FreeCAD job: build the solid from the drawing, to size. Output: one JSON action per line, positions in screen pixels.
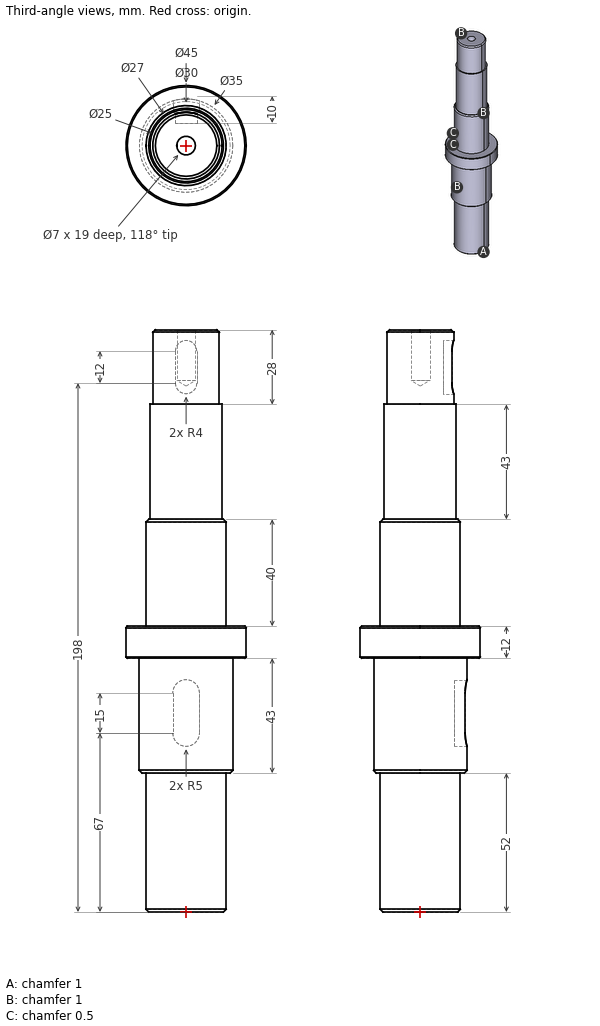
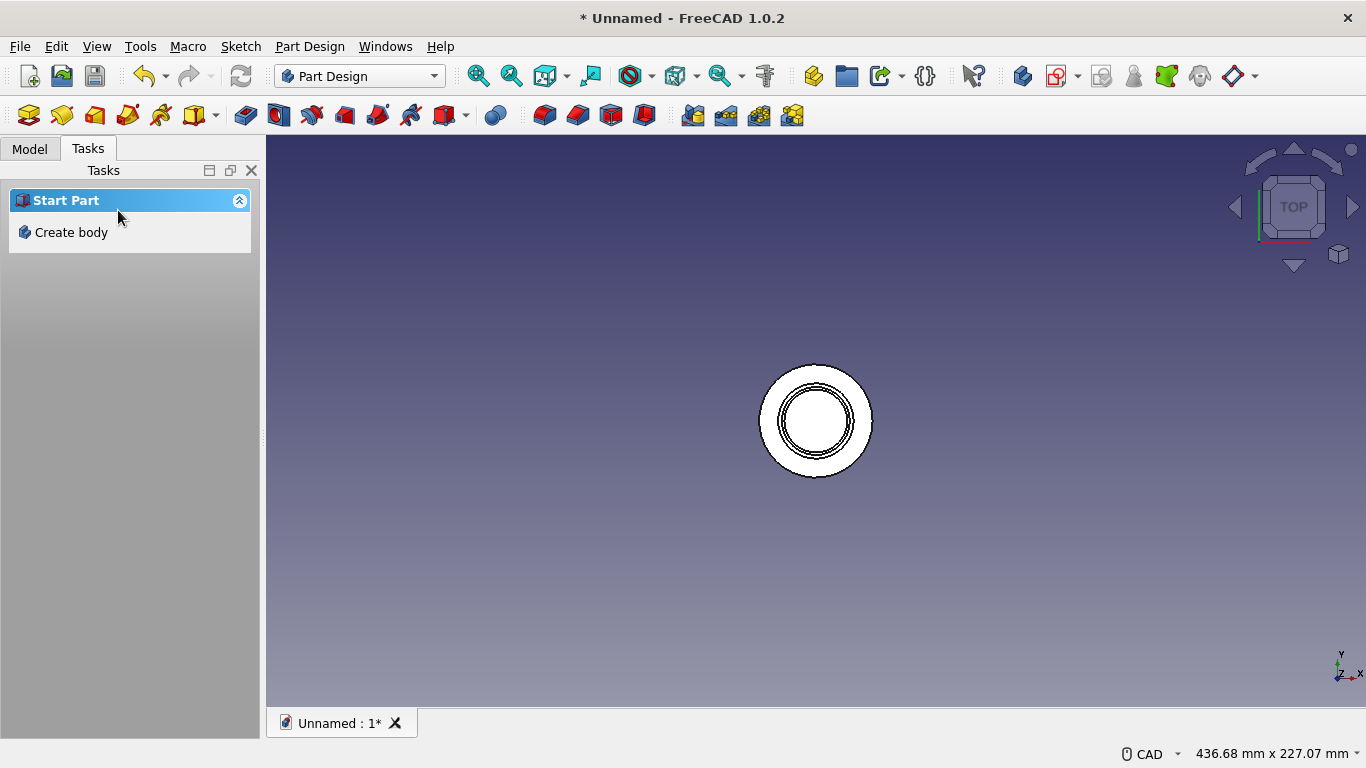
{"action": "key", "text": "1"}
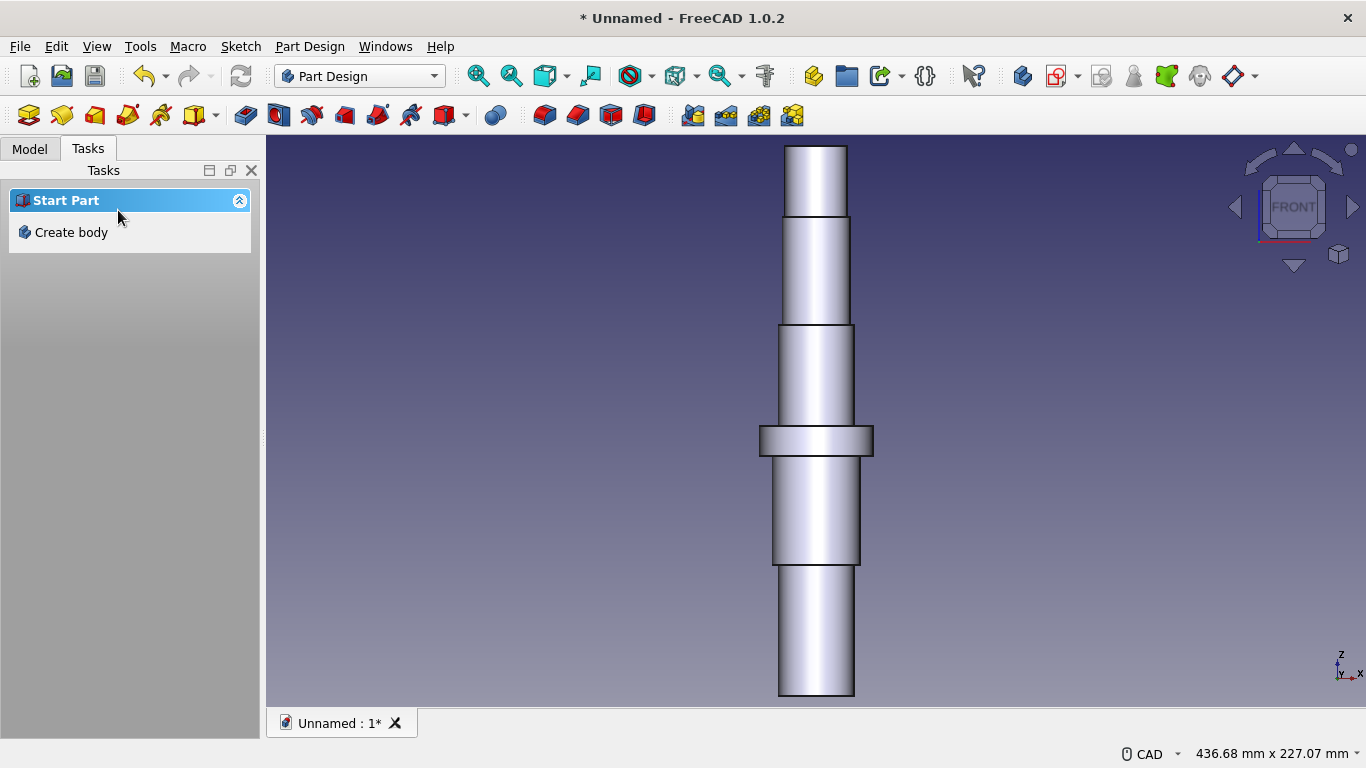
{"action": "key", "text": "3"}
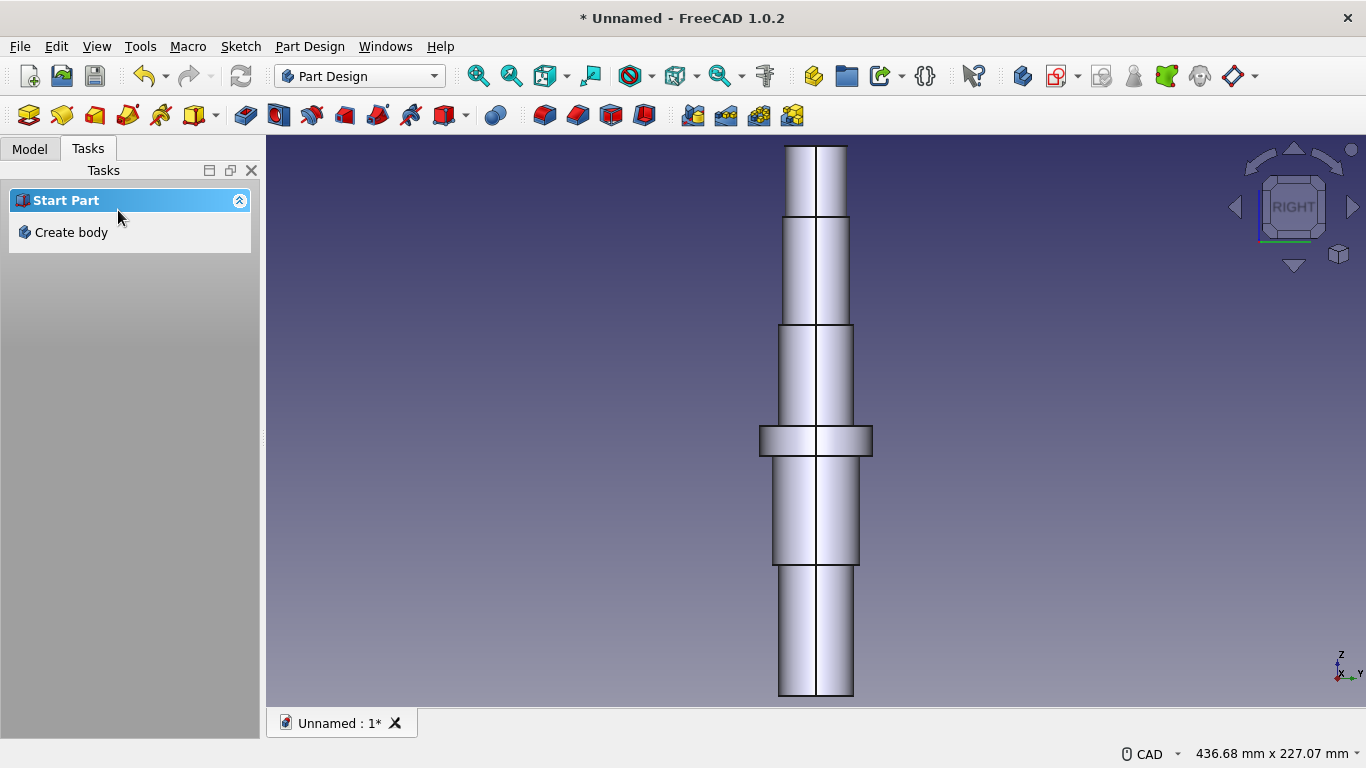
{"action": "key", "text": "5"}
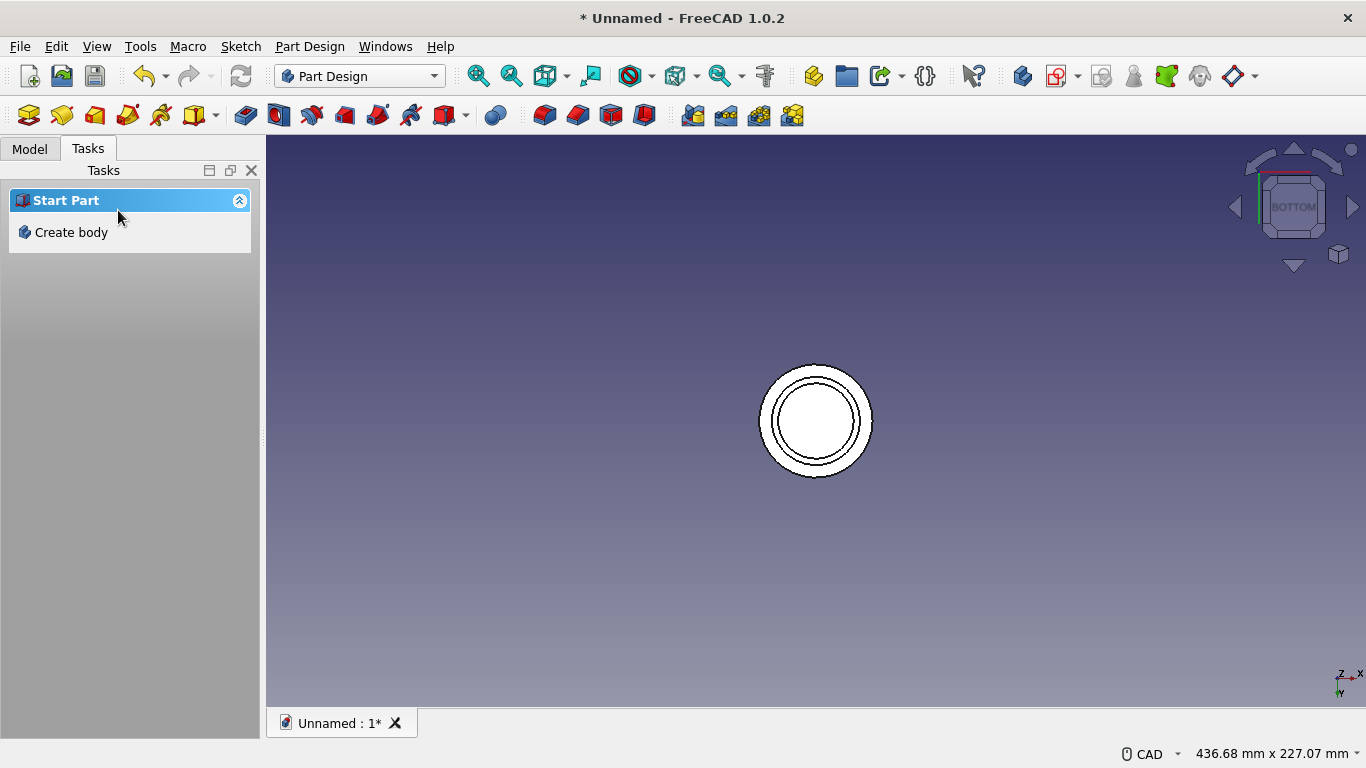
{"action": "key", "text": "v f"}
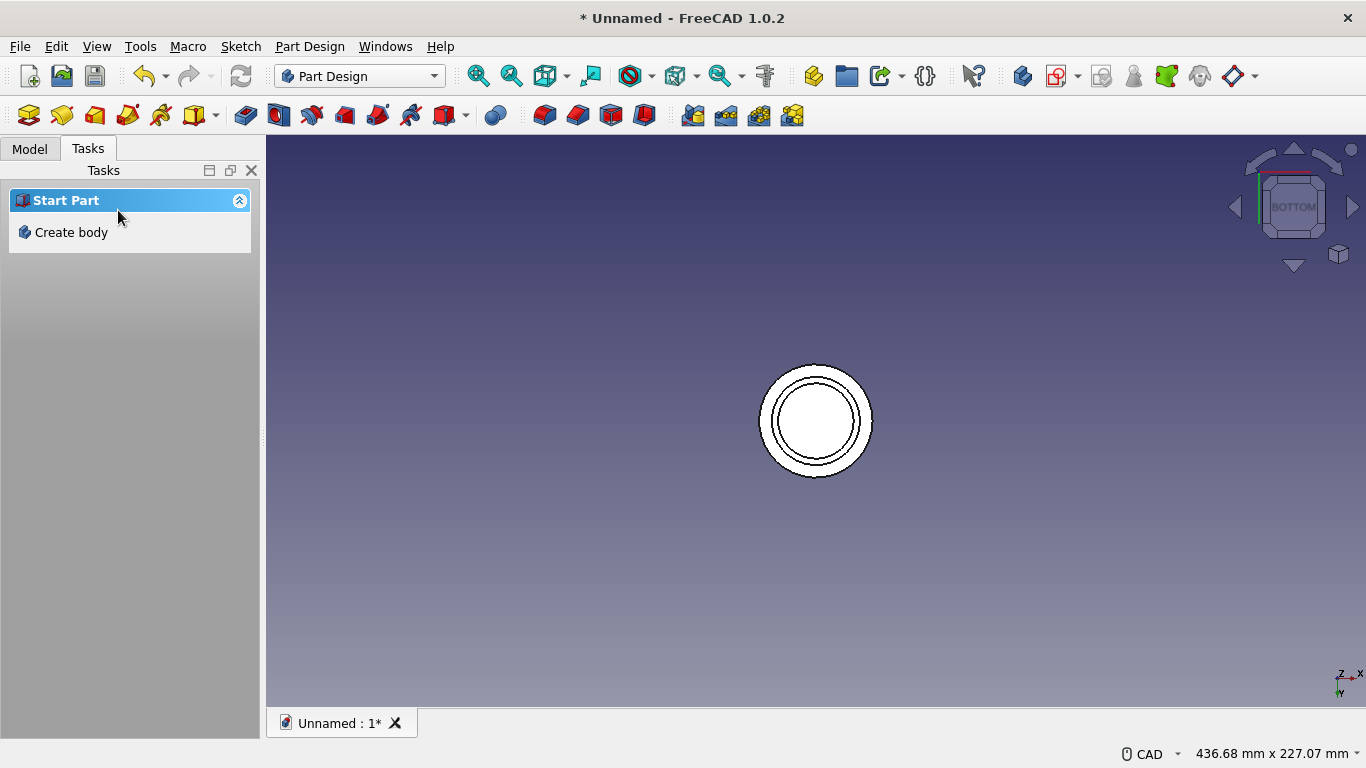
{"action": "left_click", "coordinate": [778, 420]}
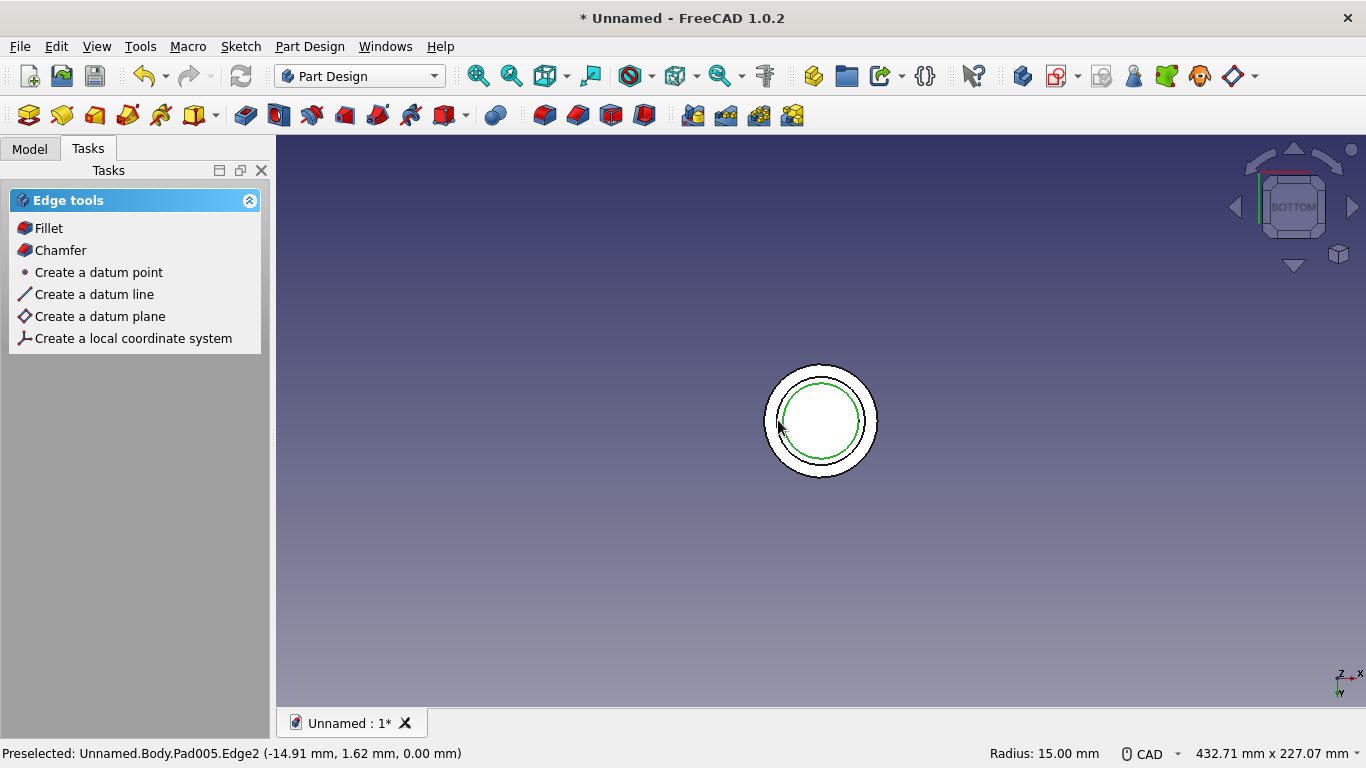
{"action": "left_click", "coordinate": [578, 116]}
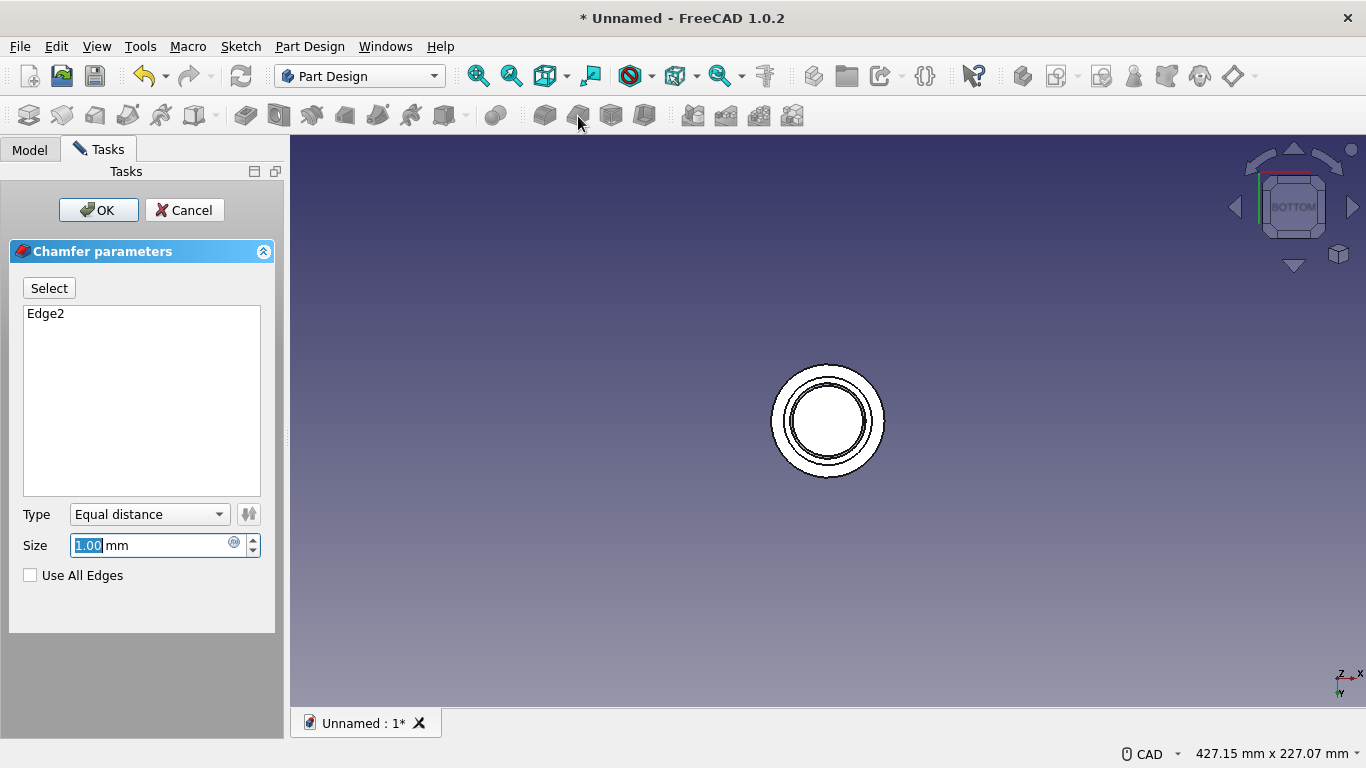
{"action": "type", "text": "1"}
{"action": "key", "text": "Tab"}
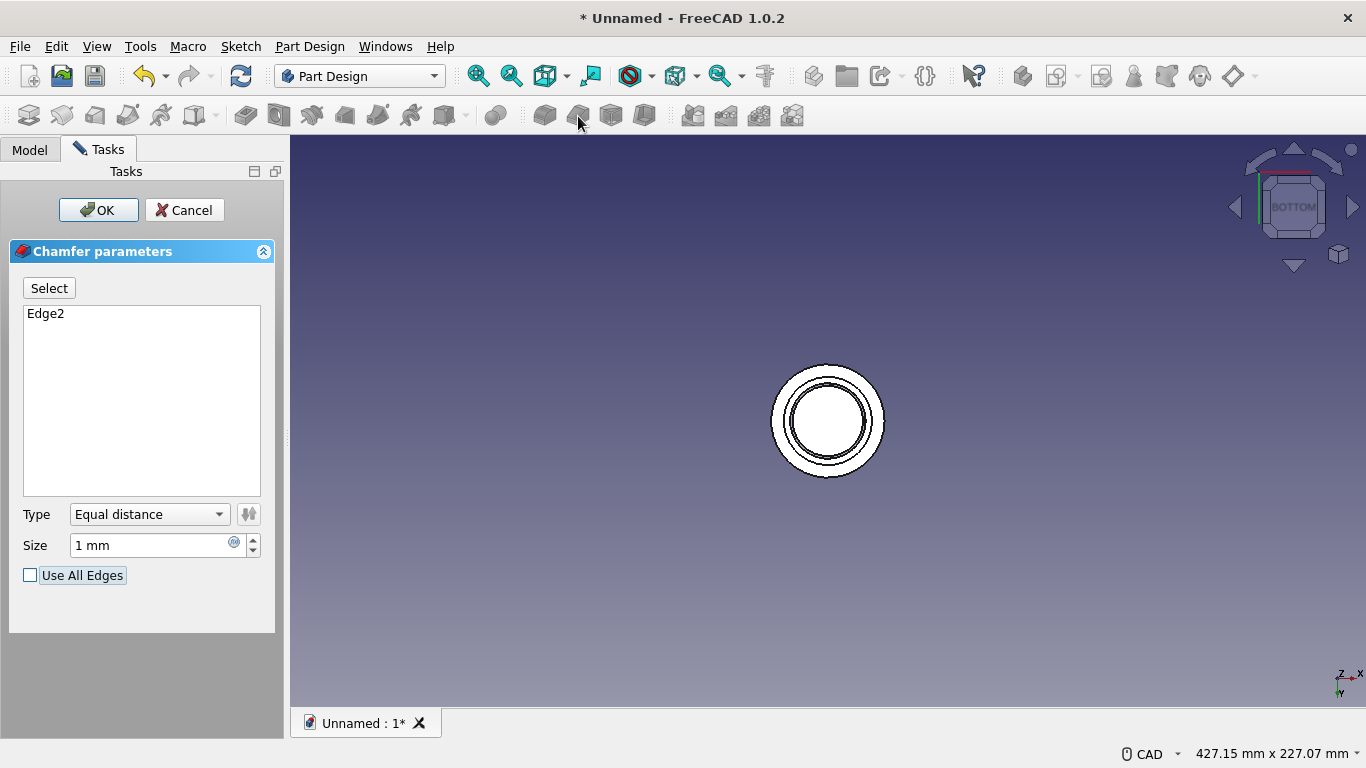
{"action": "left_click", "coordinate": [99, 210]}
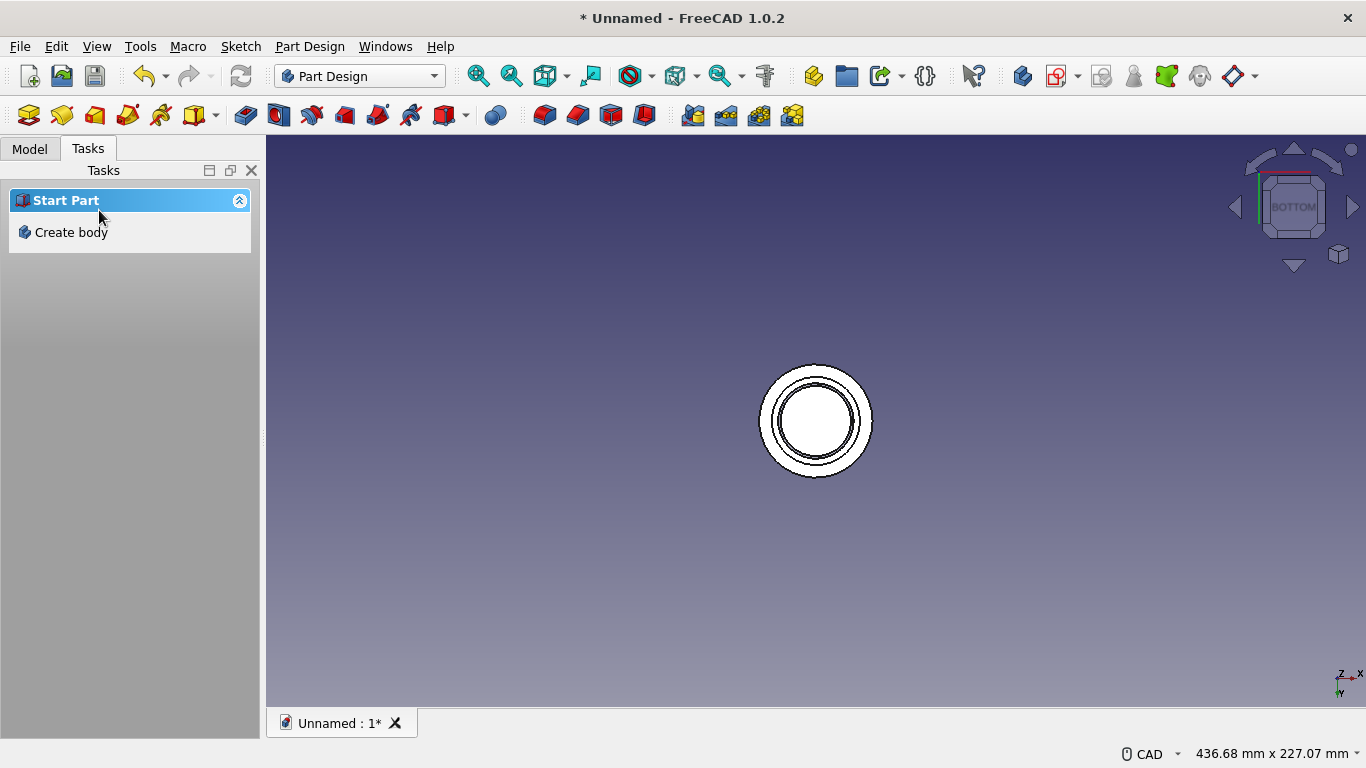
{"action": "key", "text": "v f"}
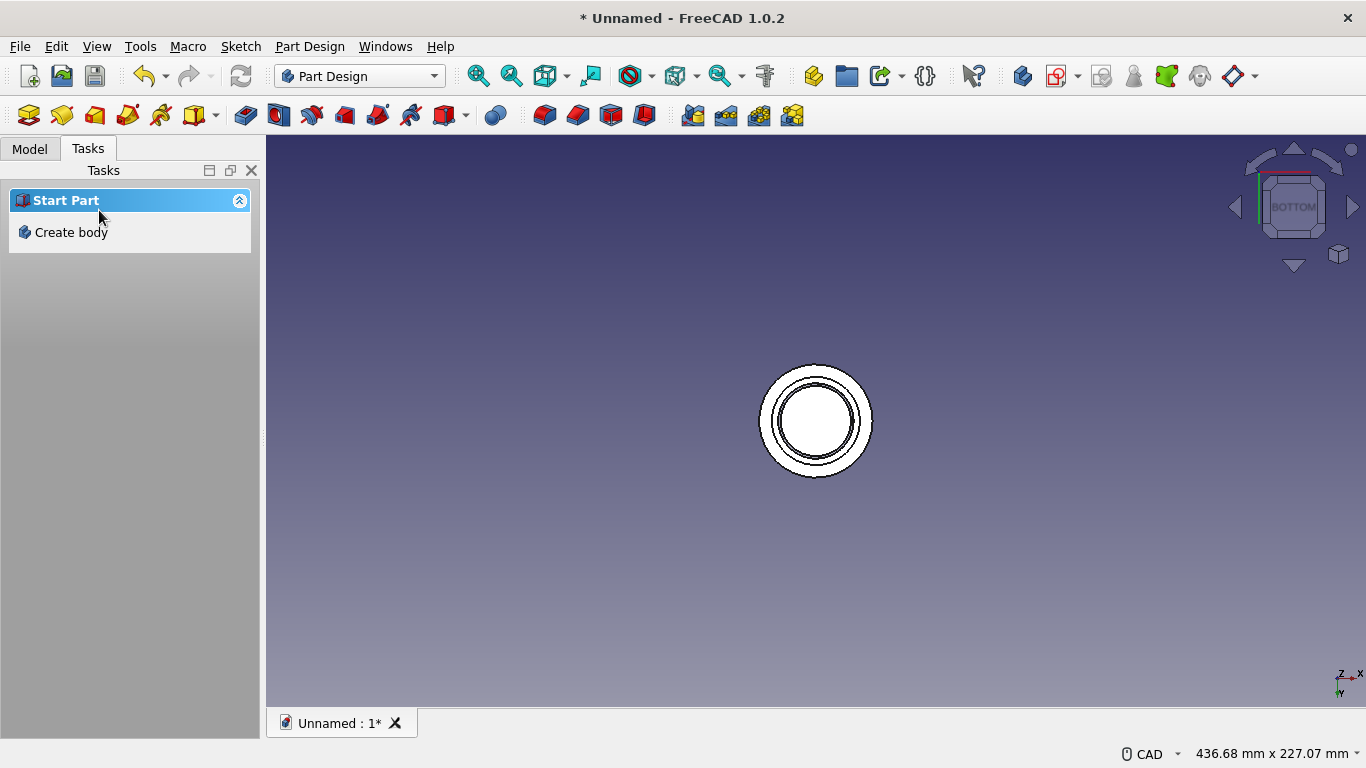
{"action": "left_click", "coordinate": [772, 420]}